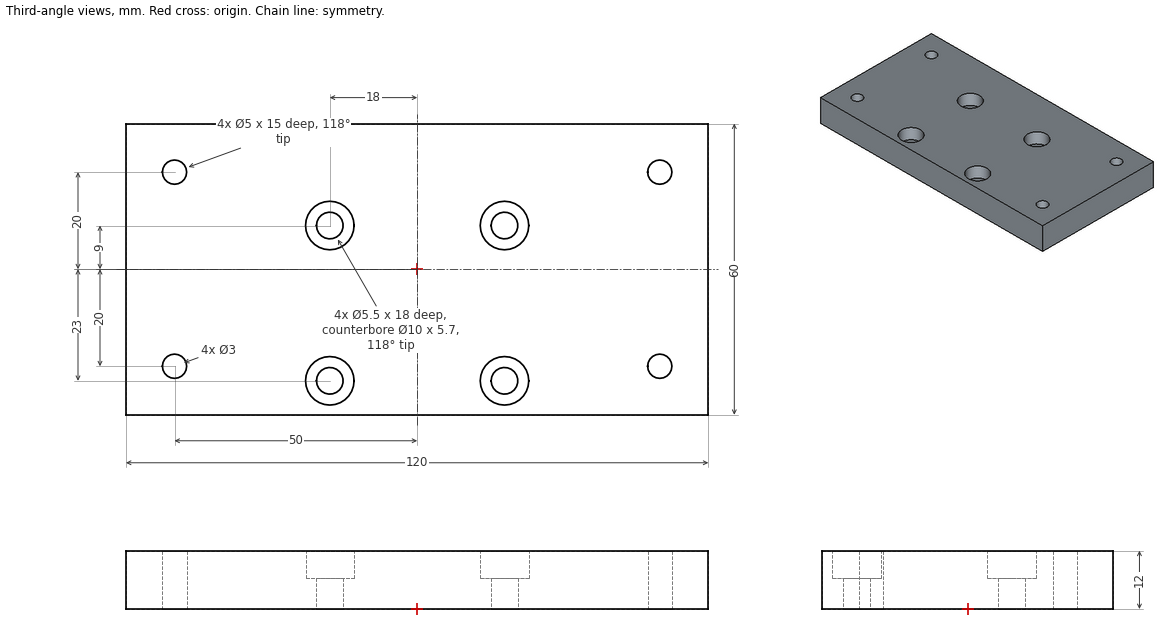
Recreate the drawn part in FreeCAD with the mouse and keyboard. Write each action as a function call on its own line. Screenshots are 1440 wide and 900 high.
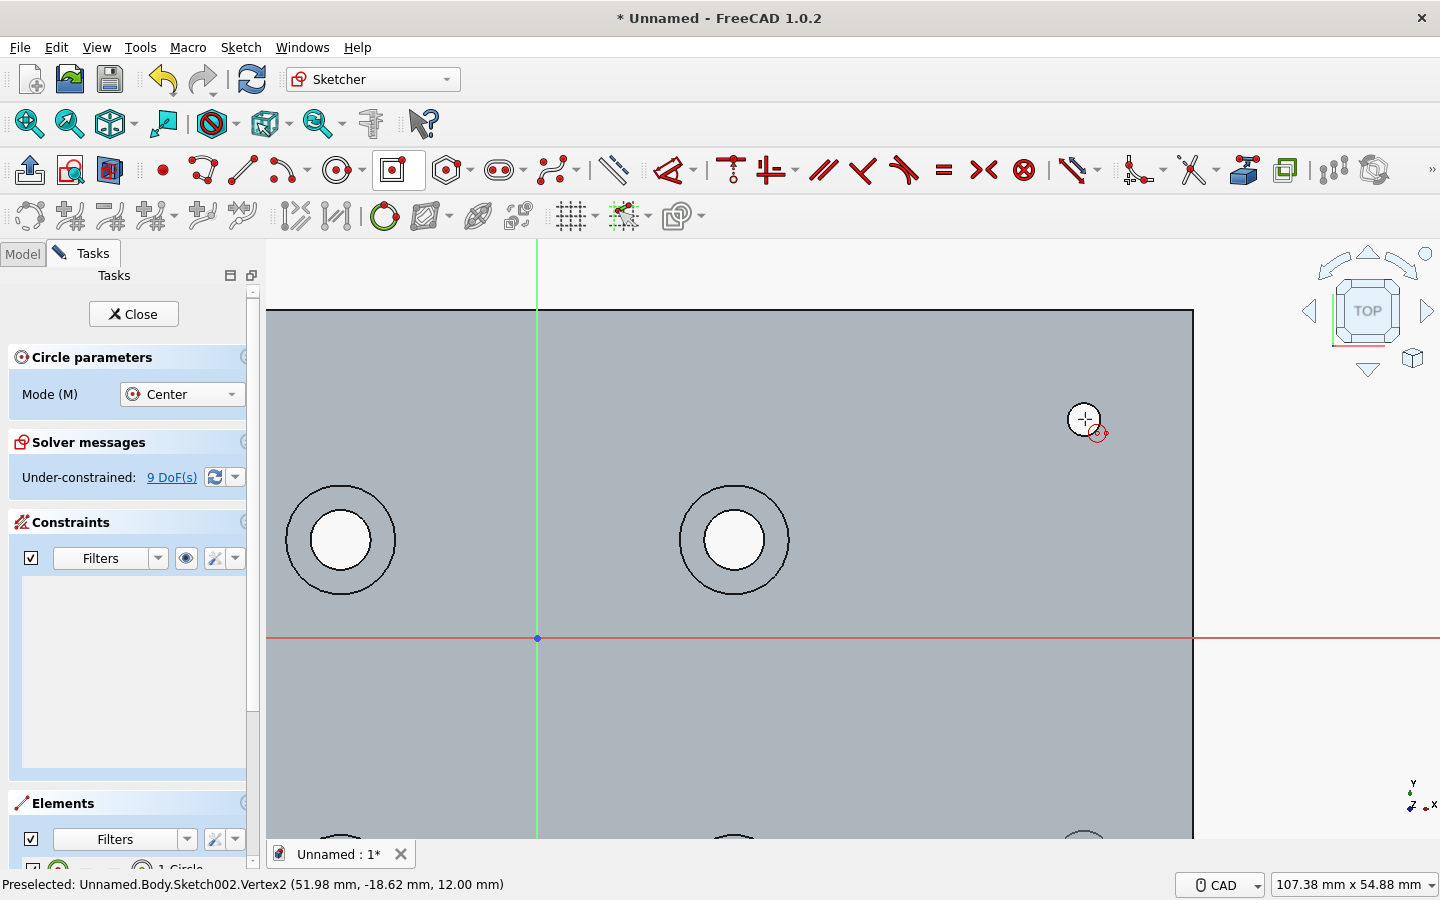
click(1084, 420)
click(1103, 400)
key(Escape)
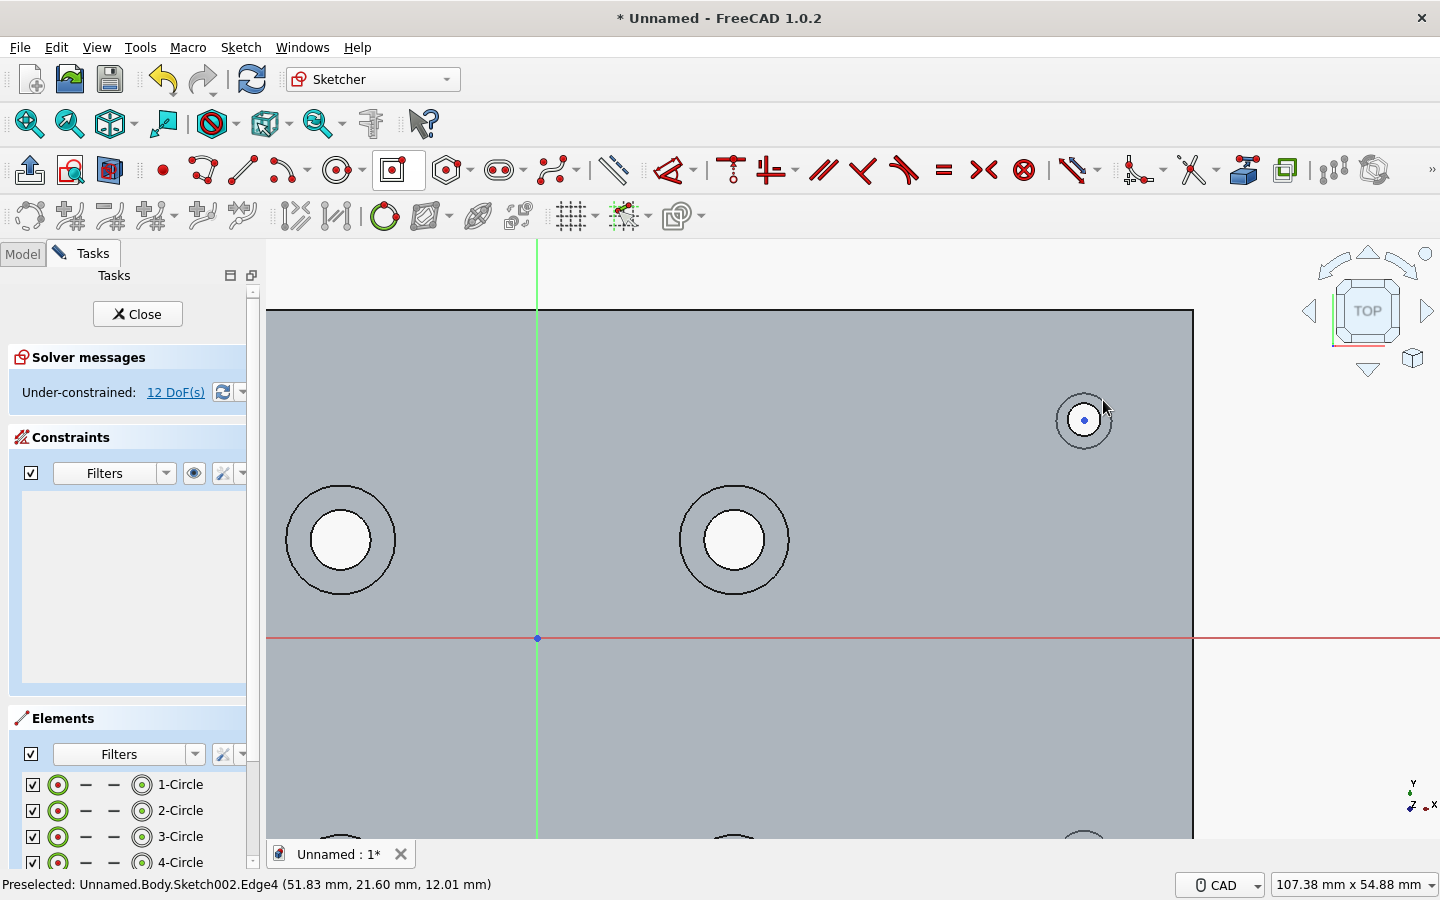
scroll(1085, 418, down, 3)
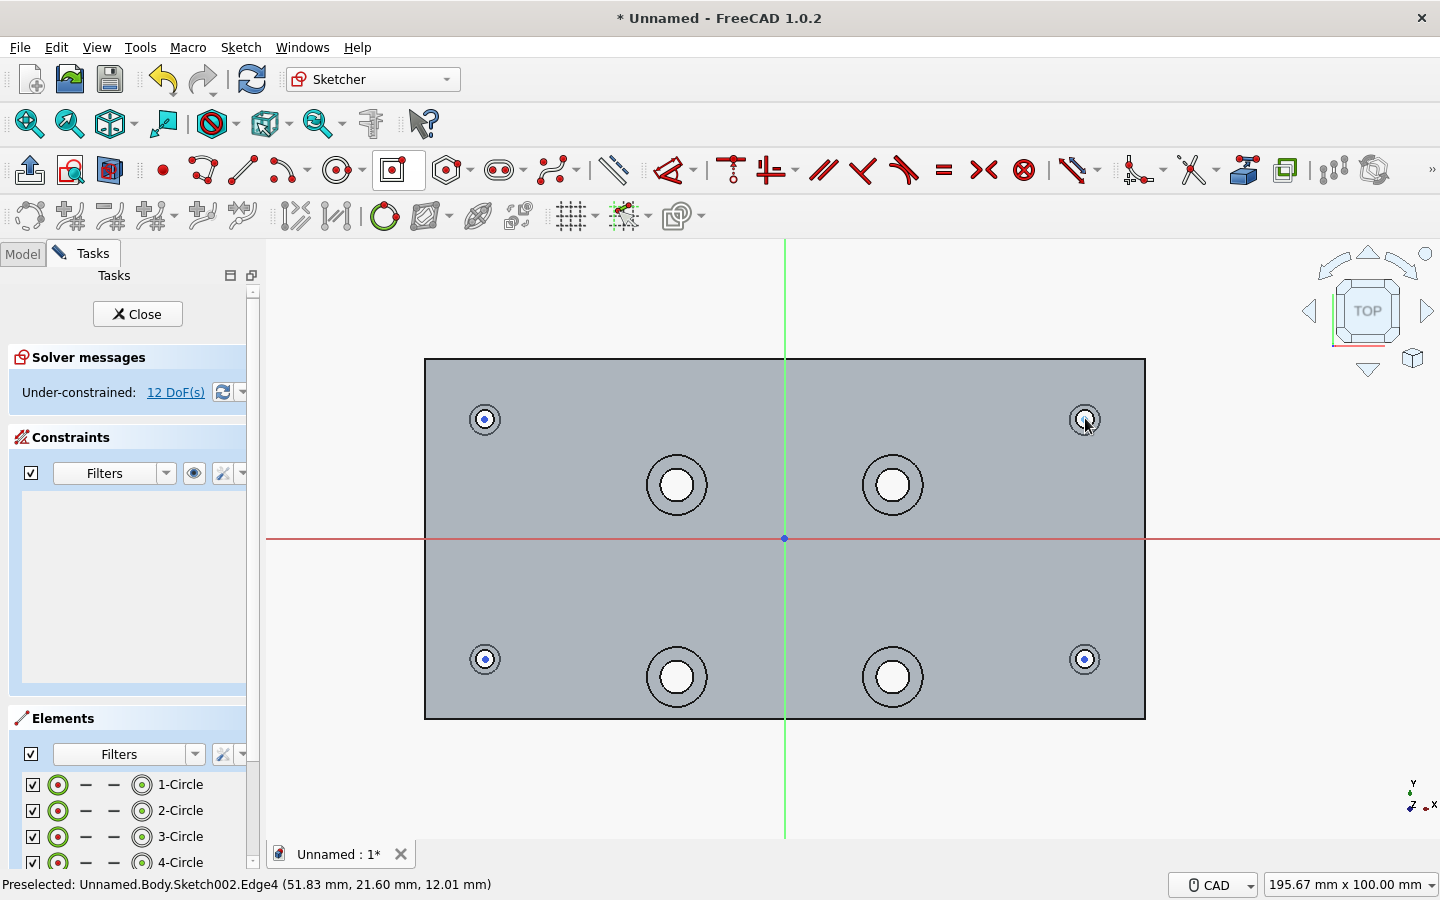
click(496, 409)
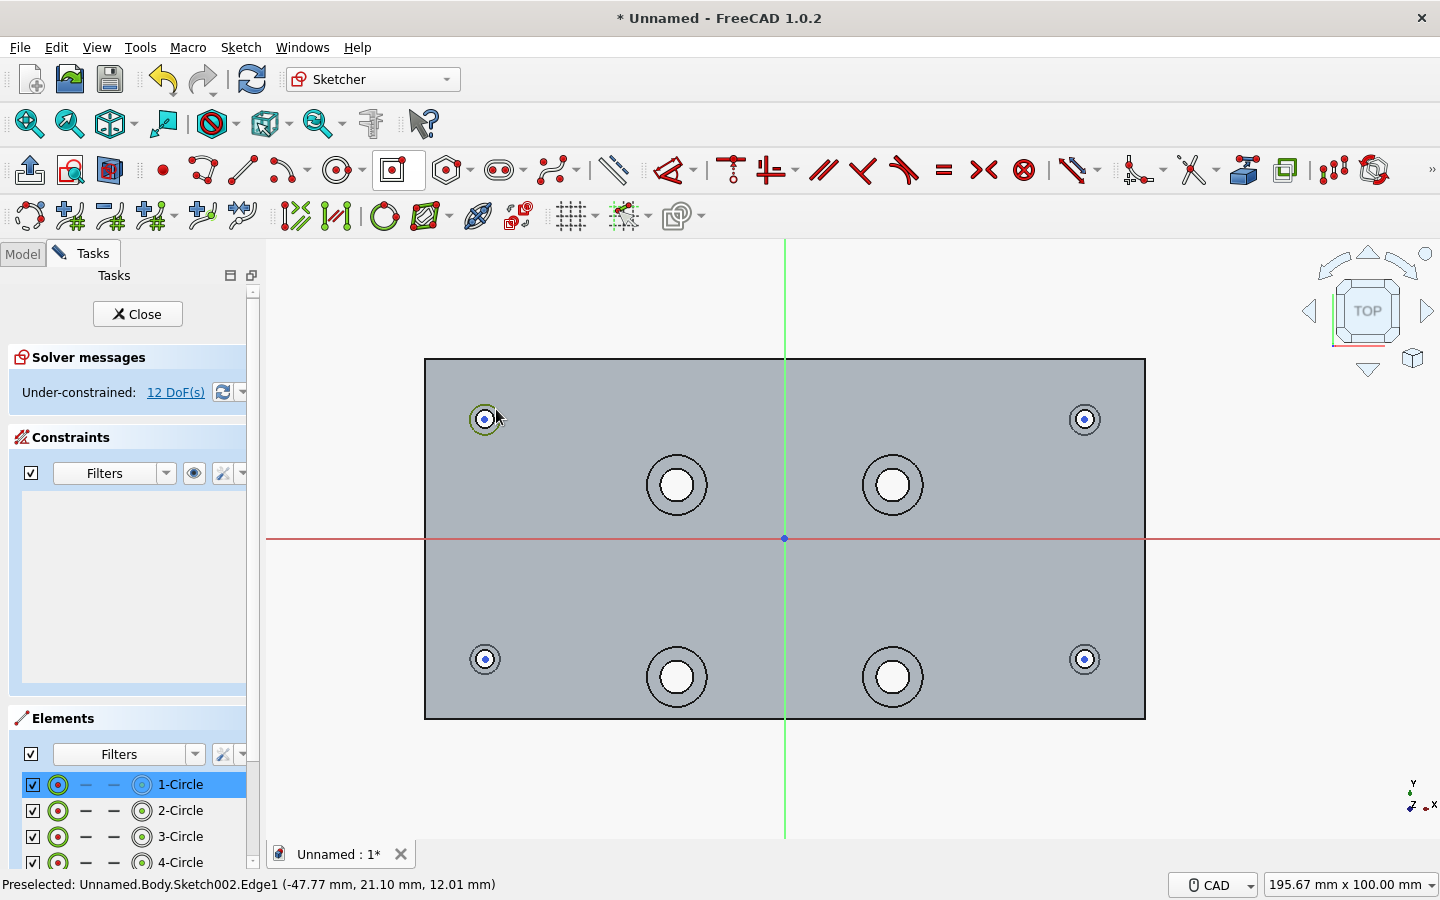
click(495, 649)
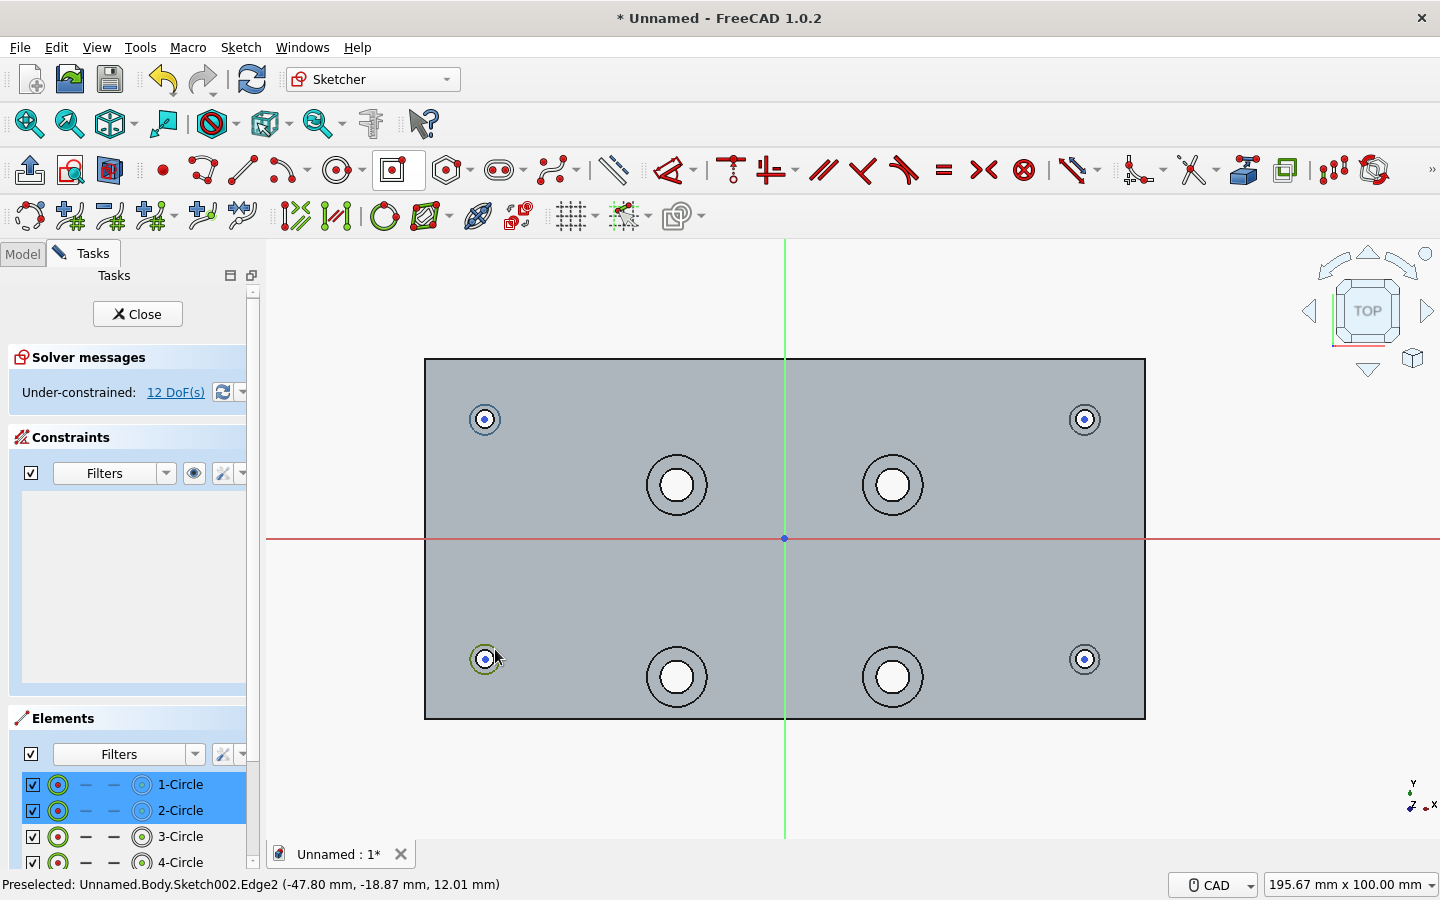
click(1095, 649)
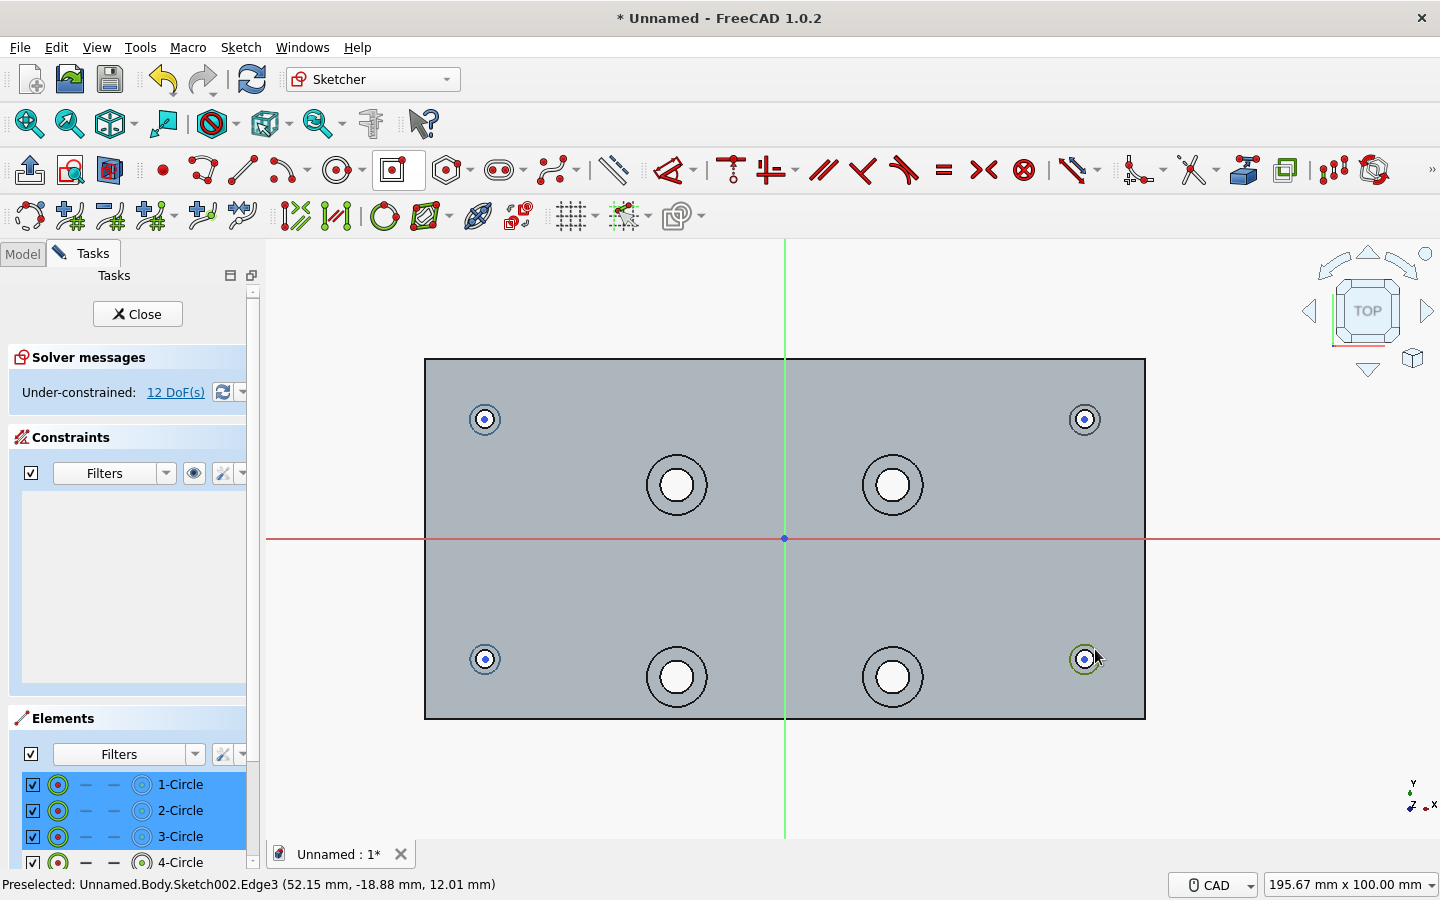
click(1095, 409)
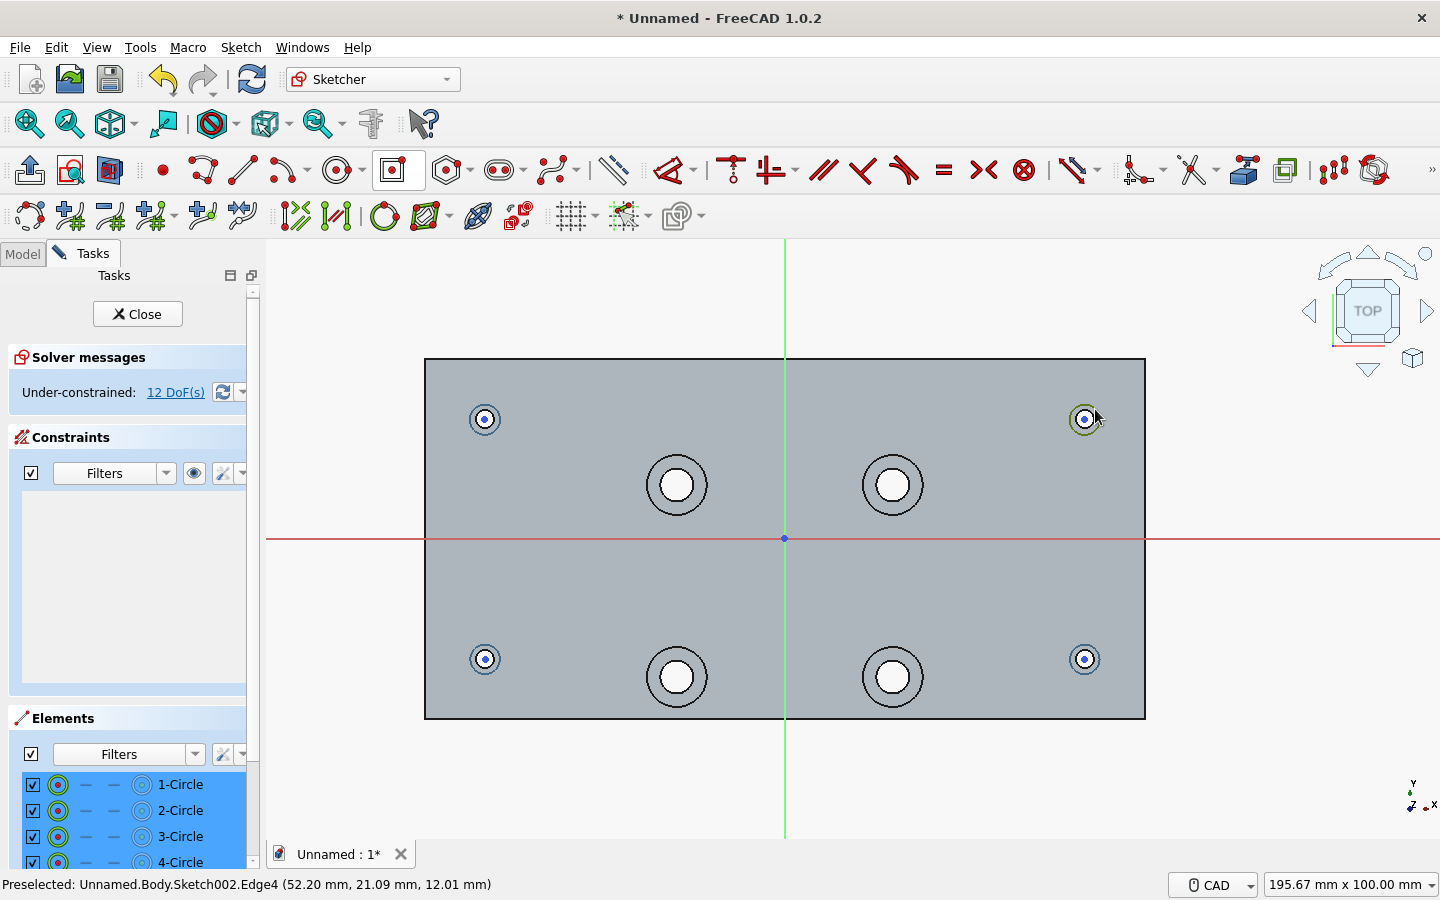
click(944, 170)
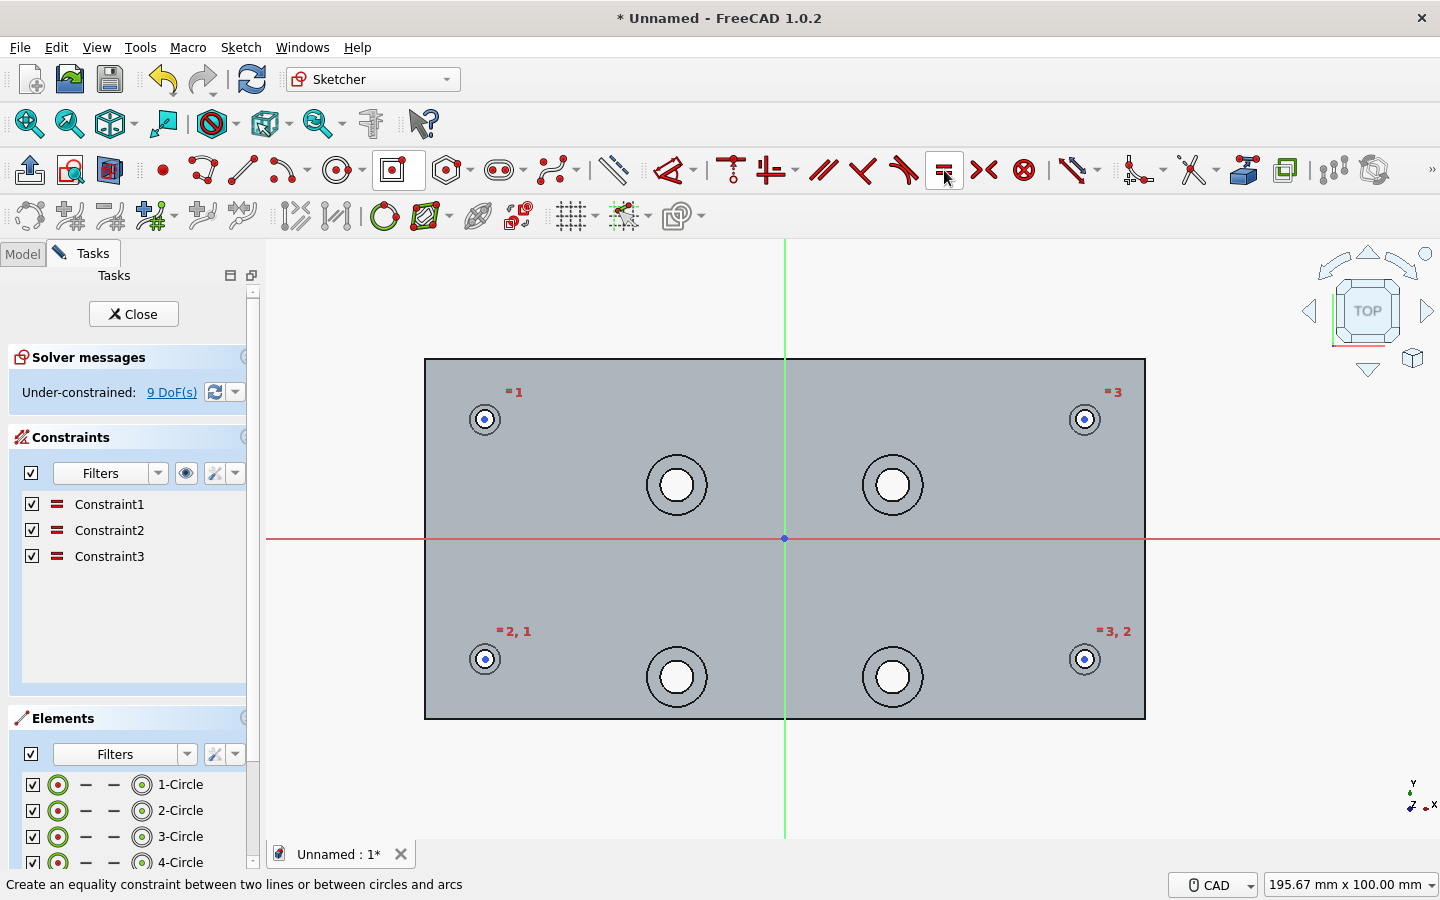
click(485, 420)